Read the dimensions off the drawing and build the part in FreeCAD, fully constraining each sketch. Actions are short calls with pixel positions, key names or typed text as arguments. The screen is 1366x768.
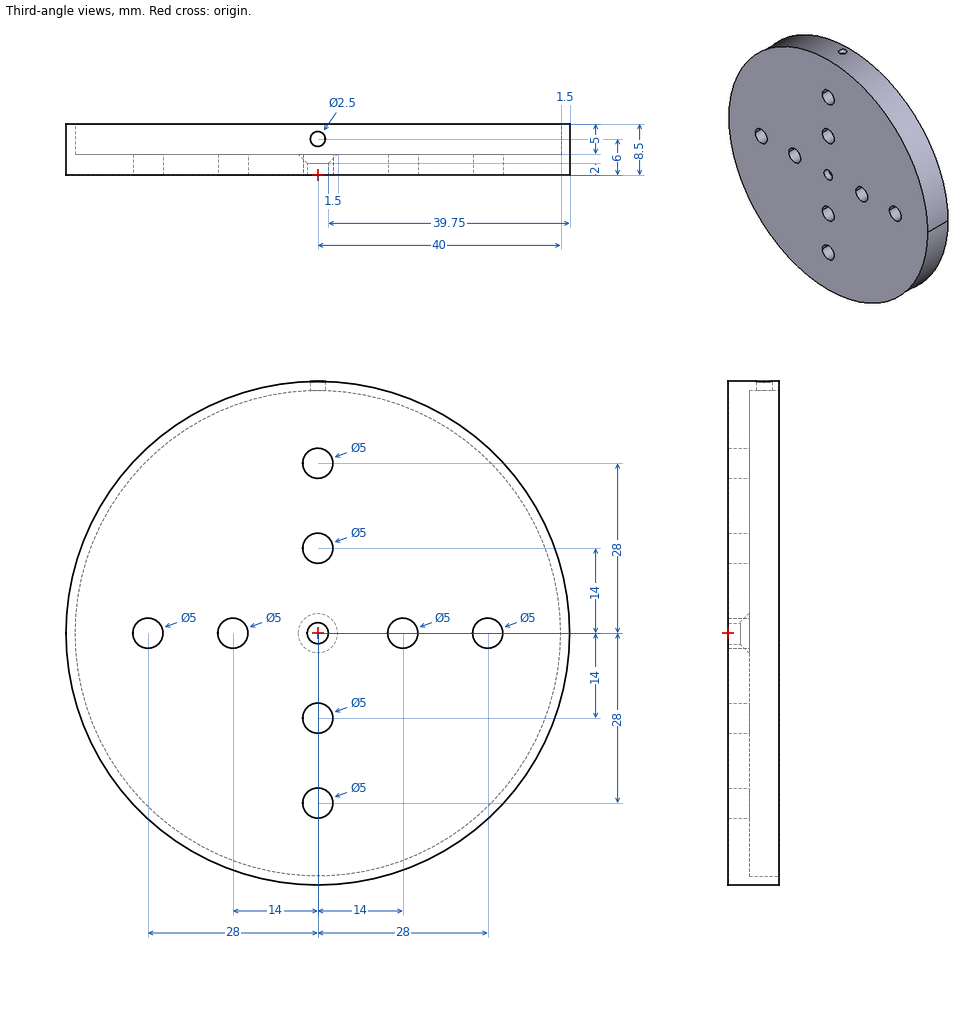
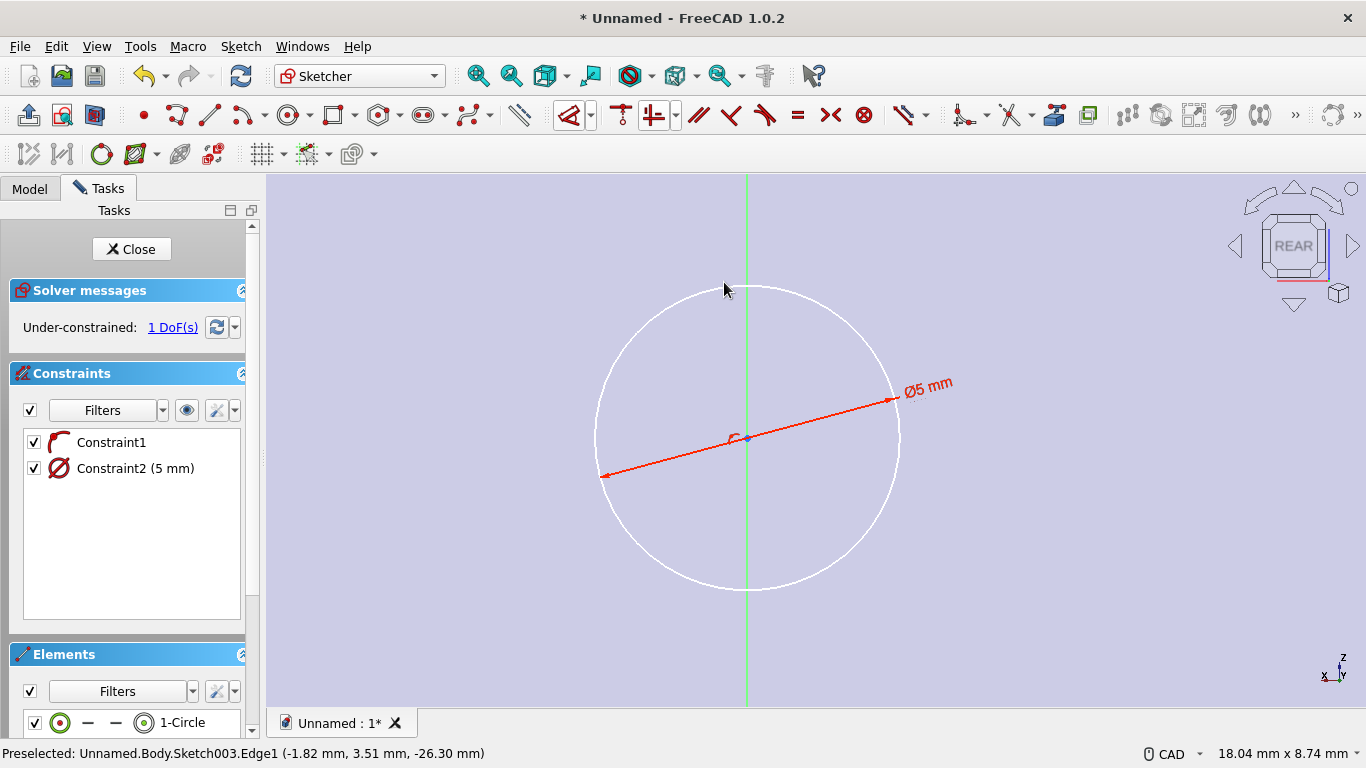
click(747, 438)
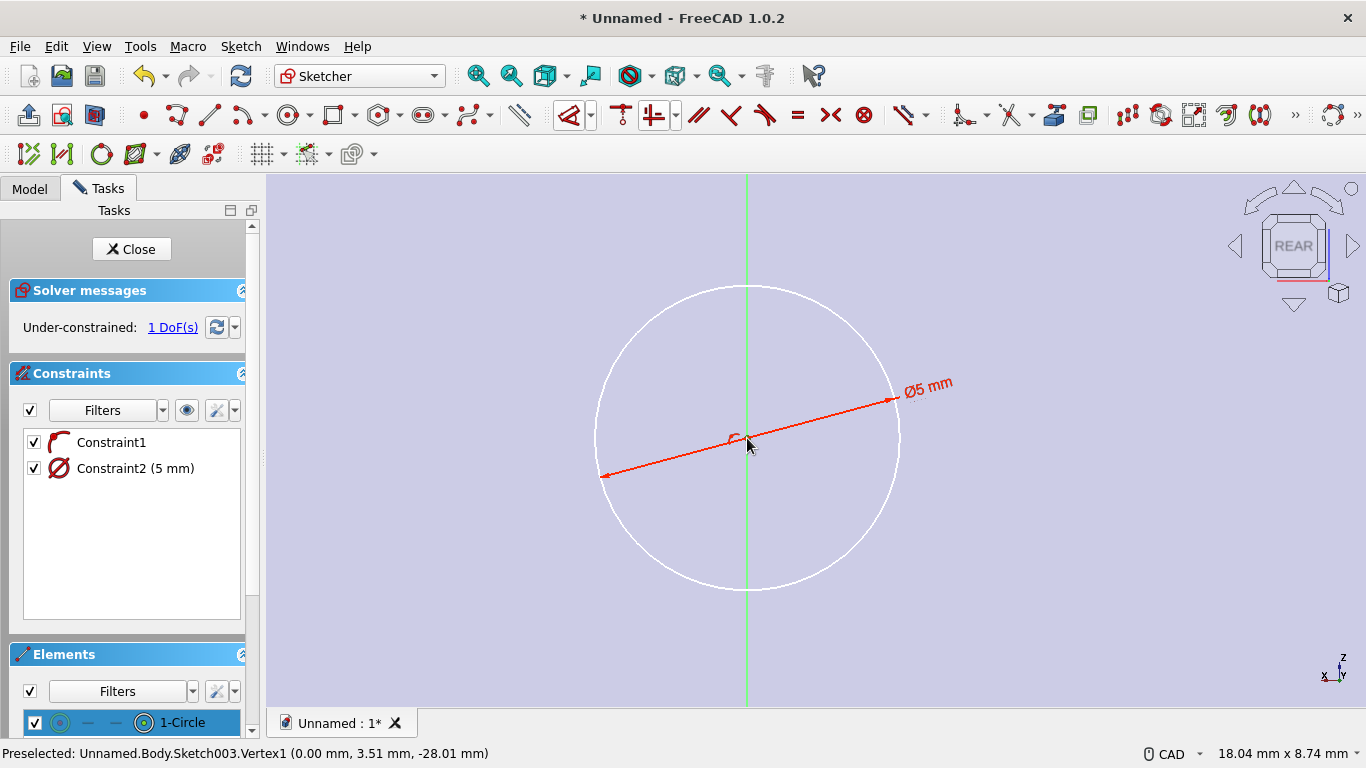
click(590, 116)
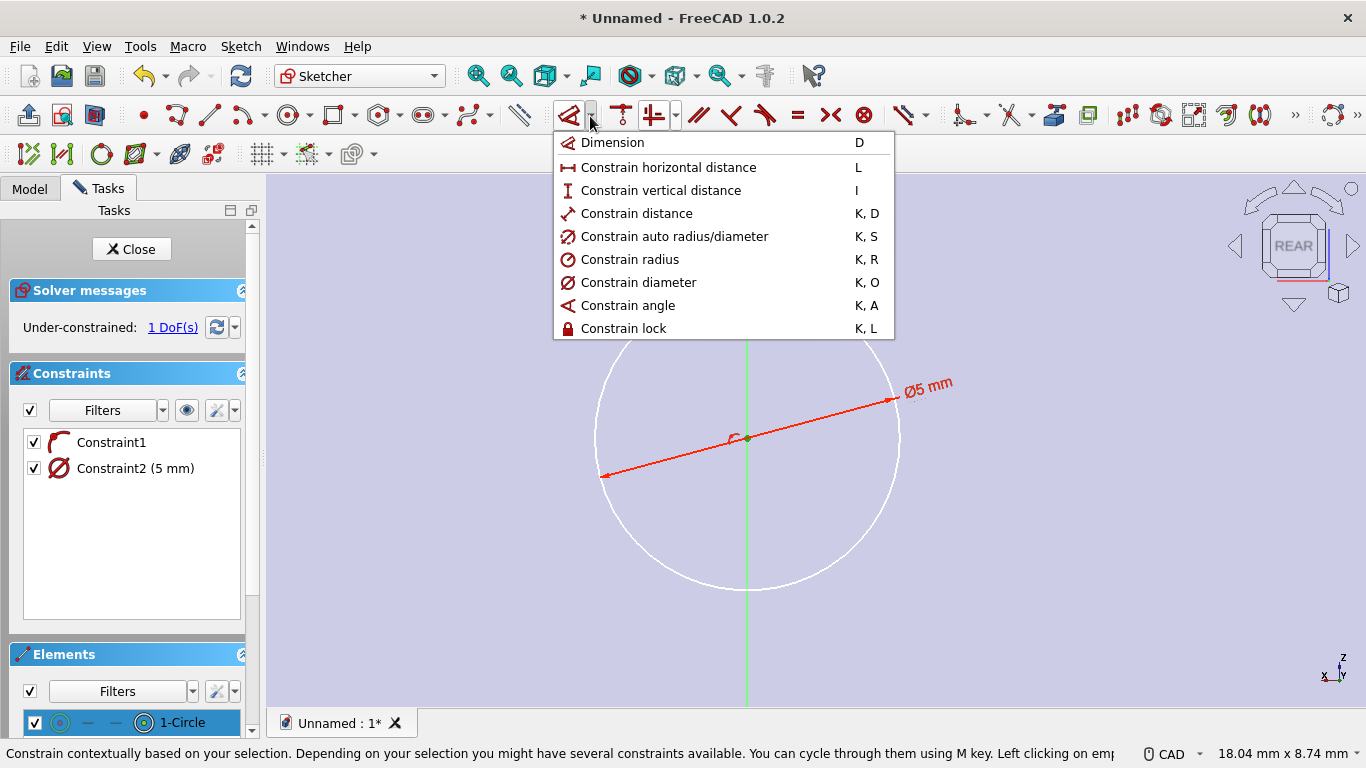
click(724, 190)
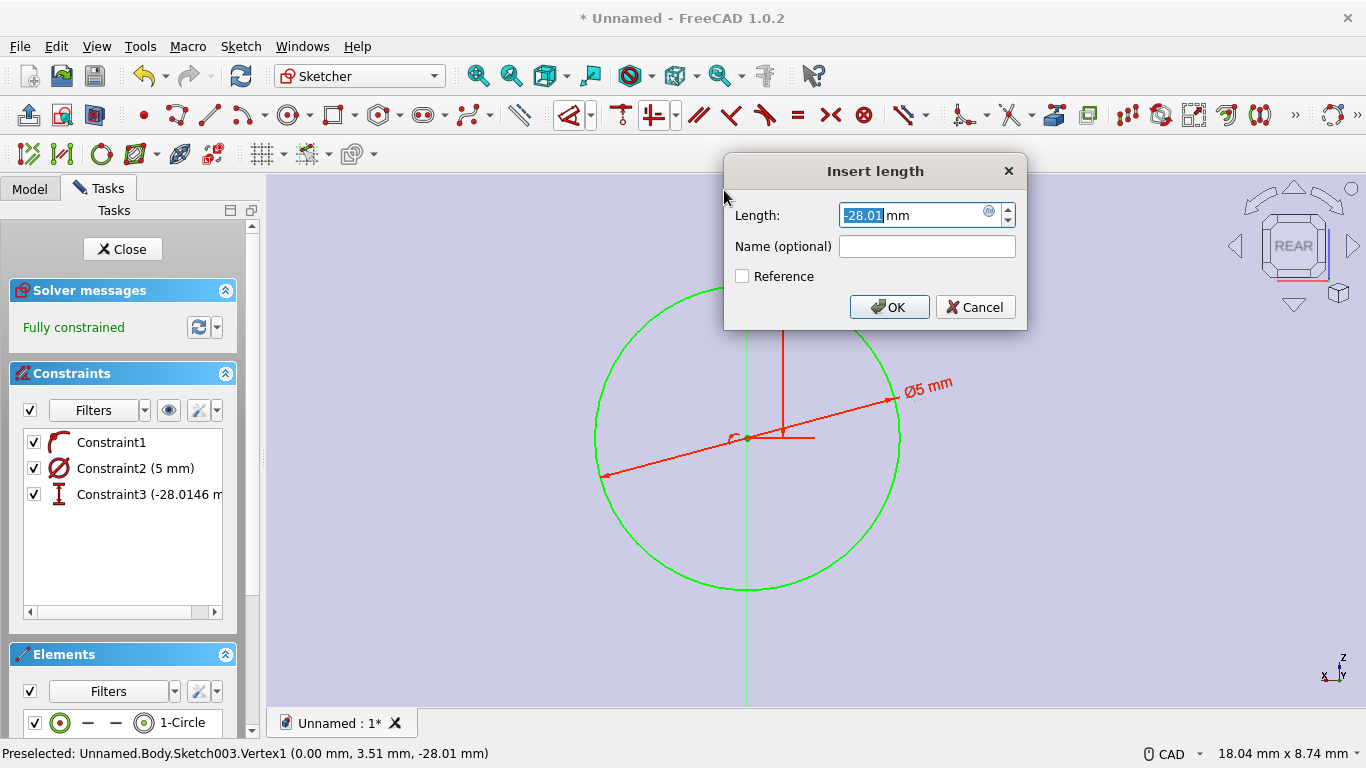
text(-28)
key(Return)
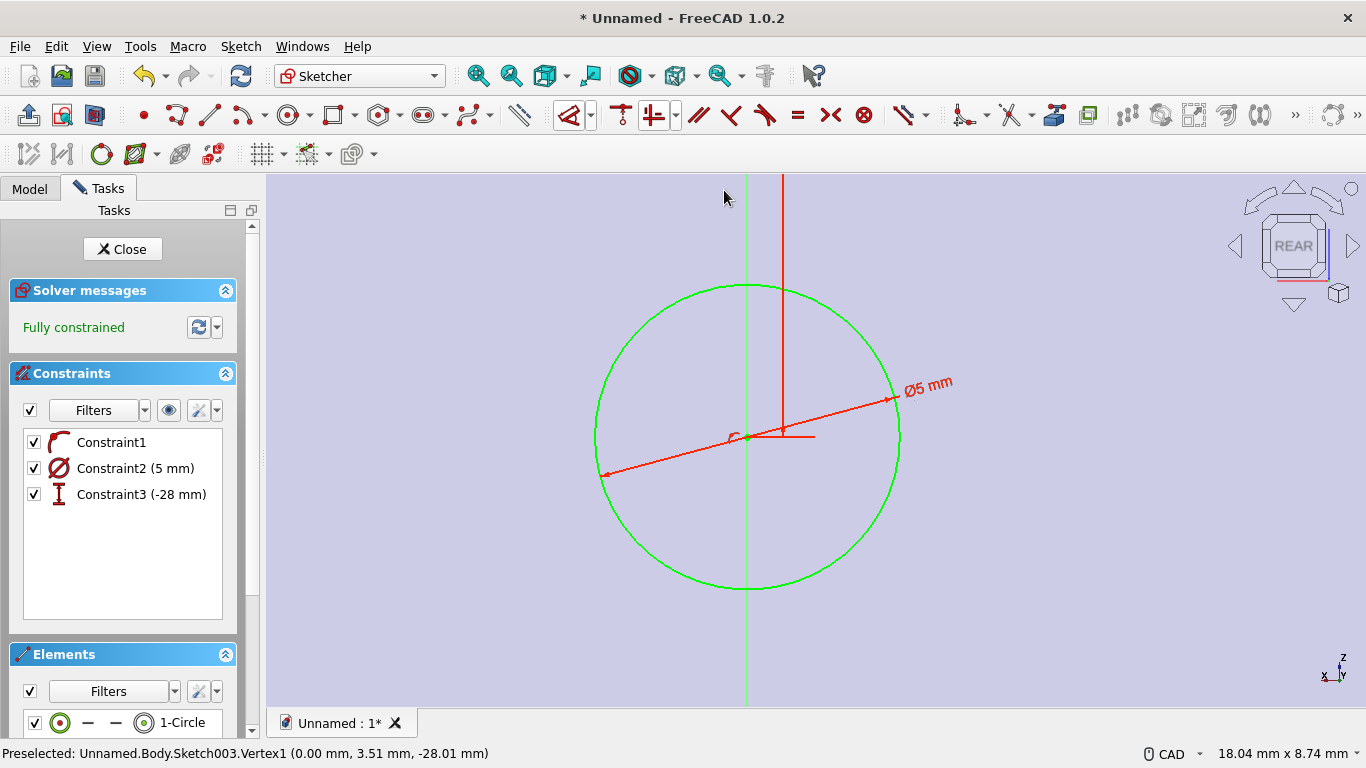
click(123, 249)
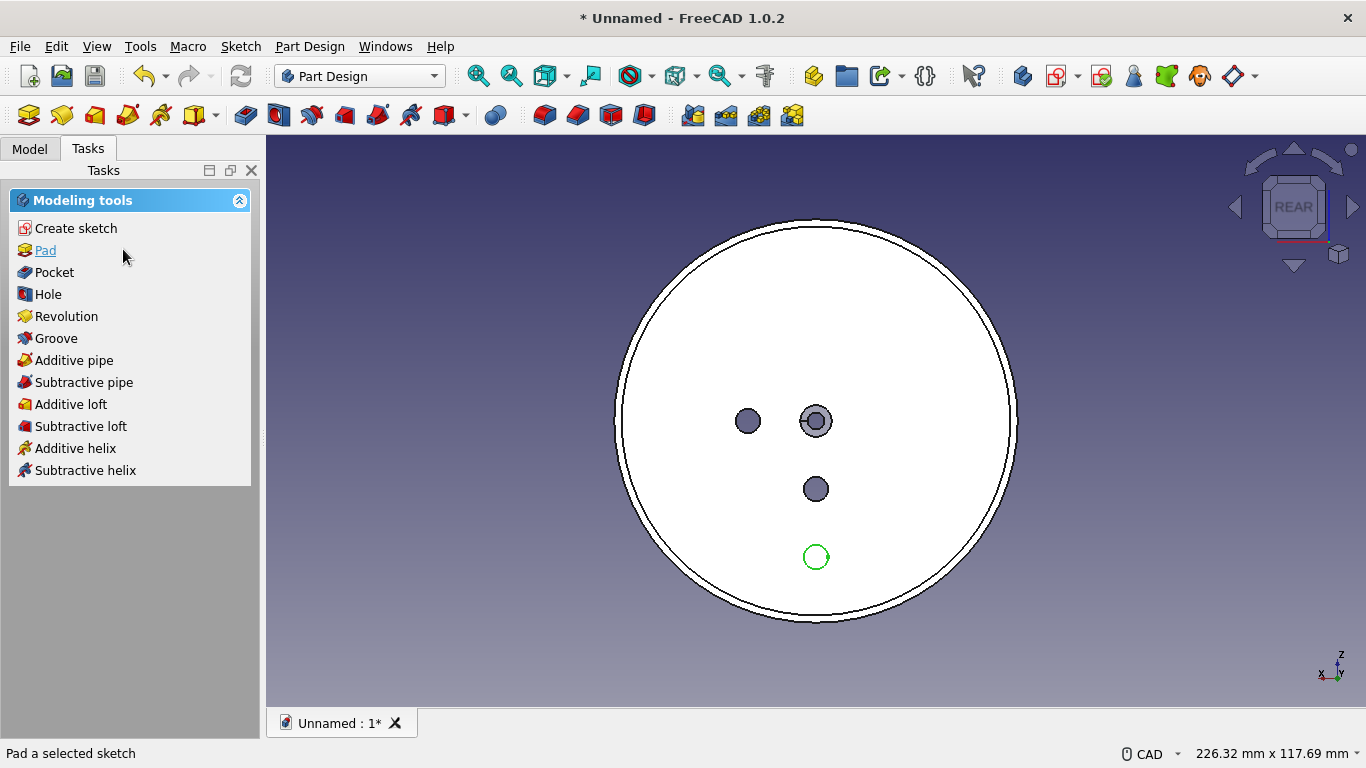
click(246, 116)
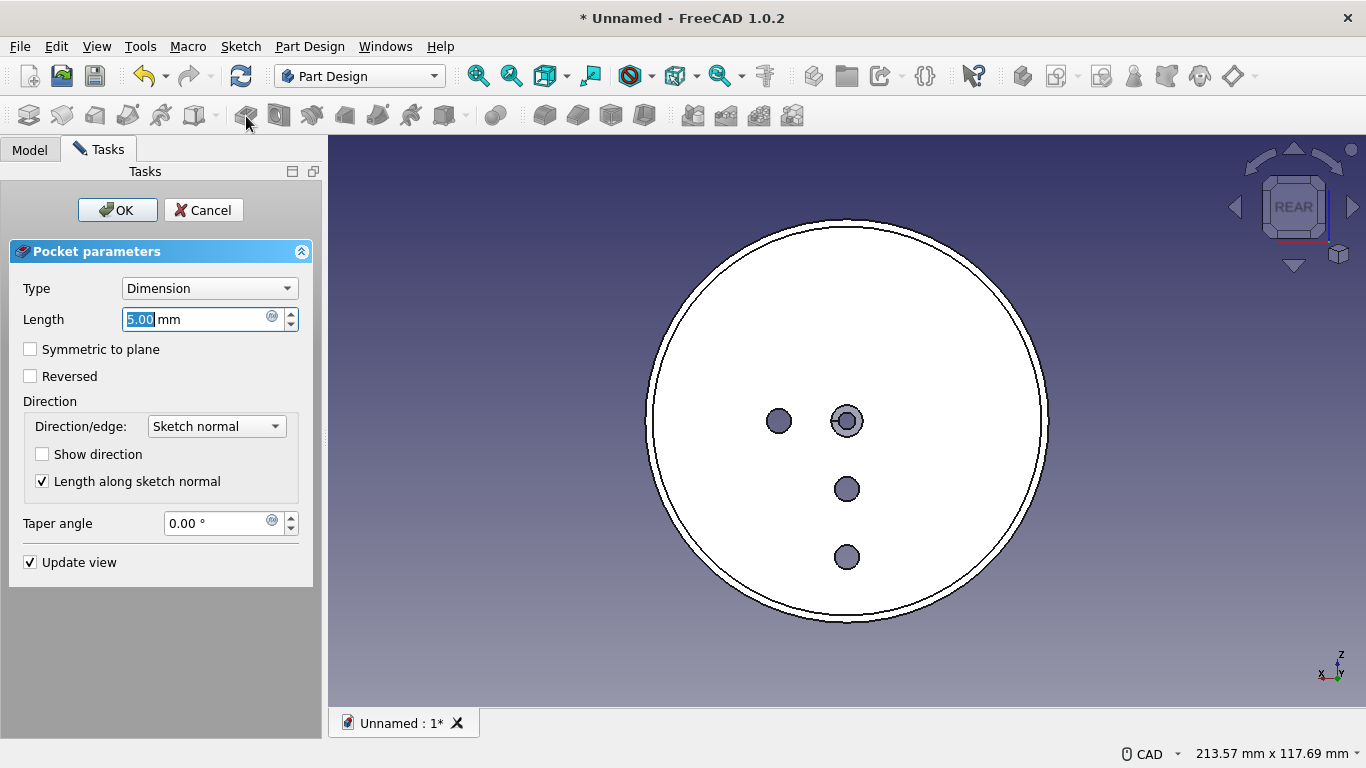
click(210, 288)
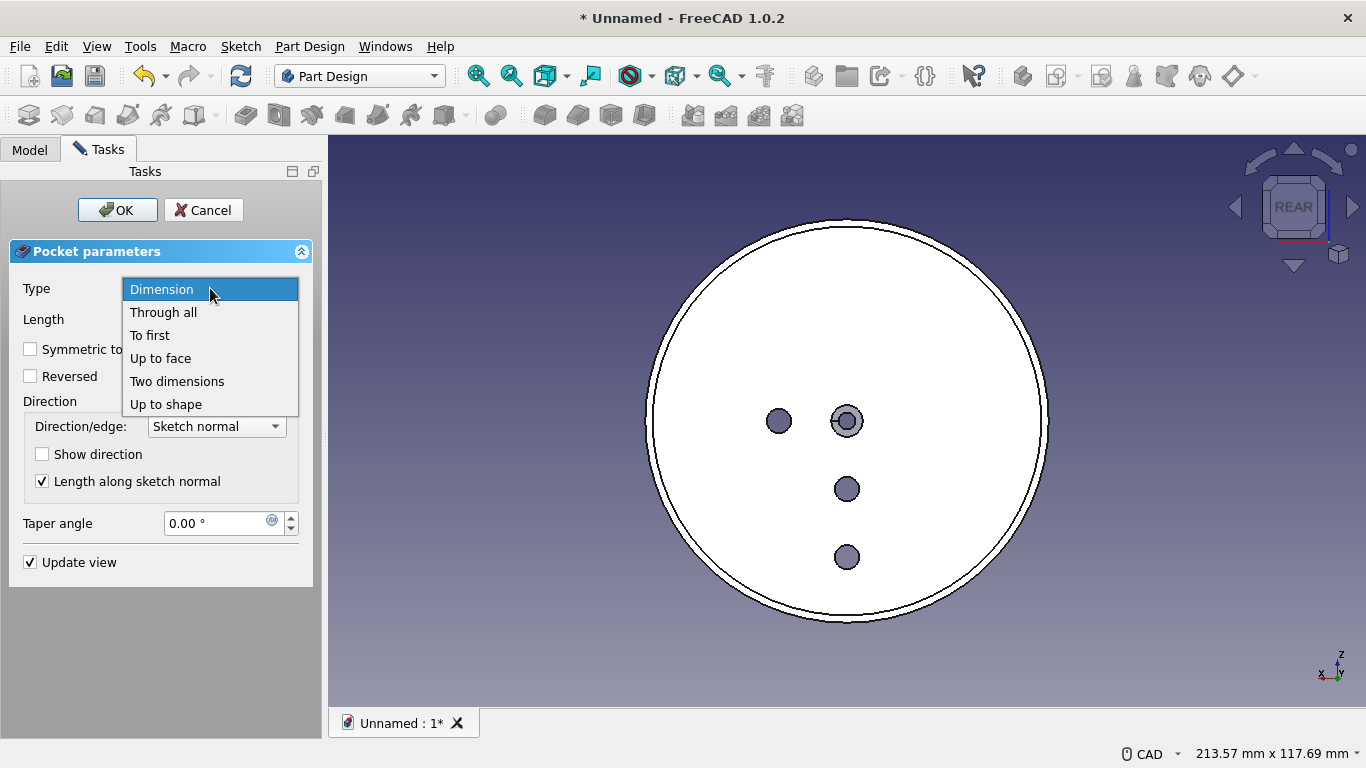
click(208, 336)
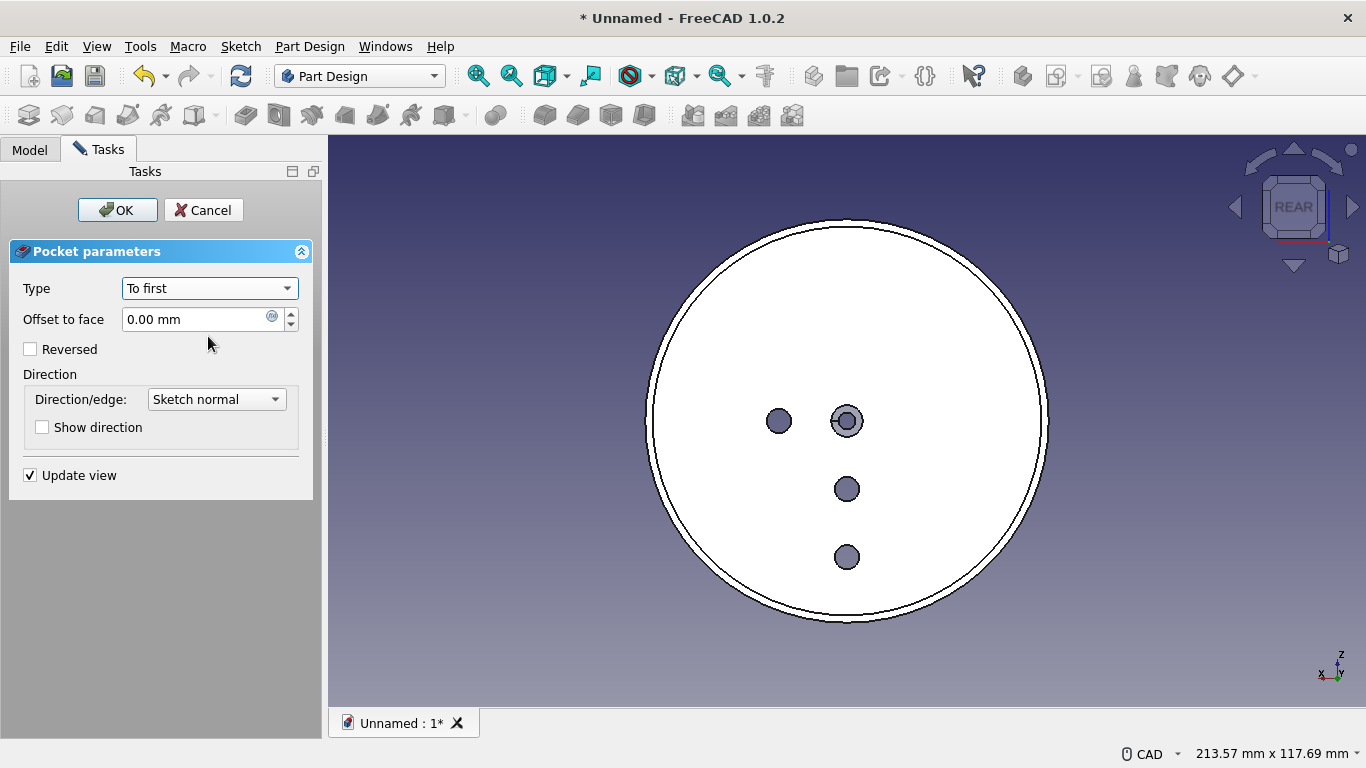
click(118, 210)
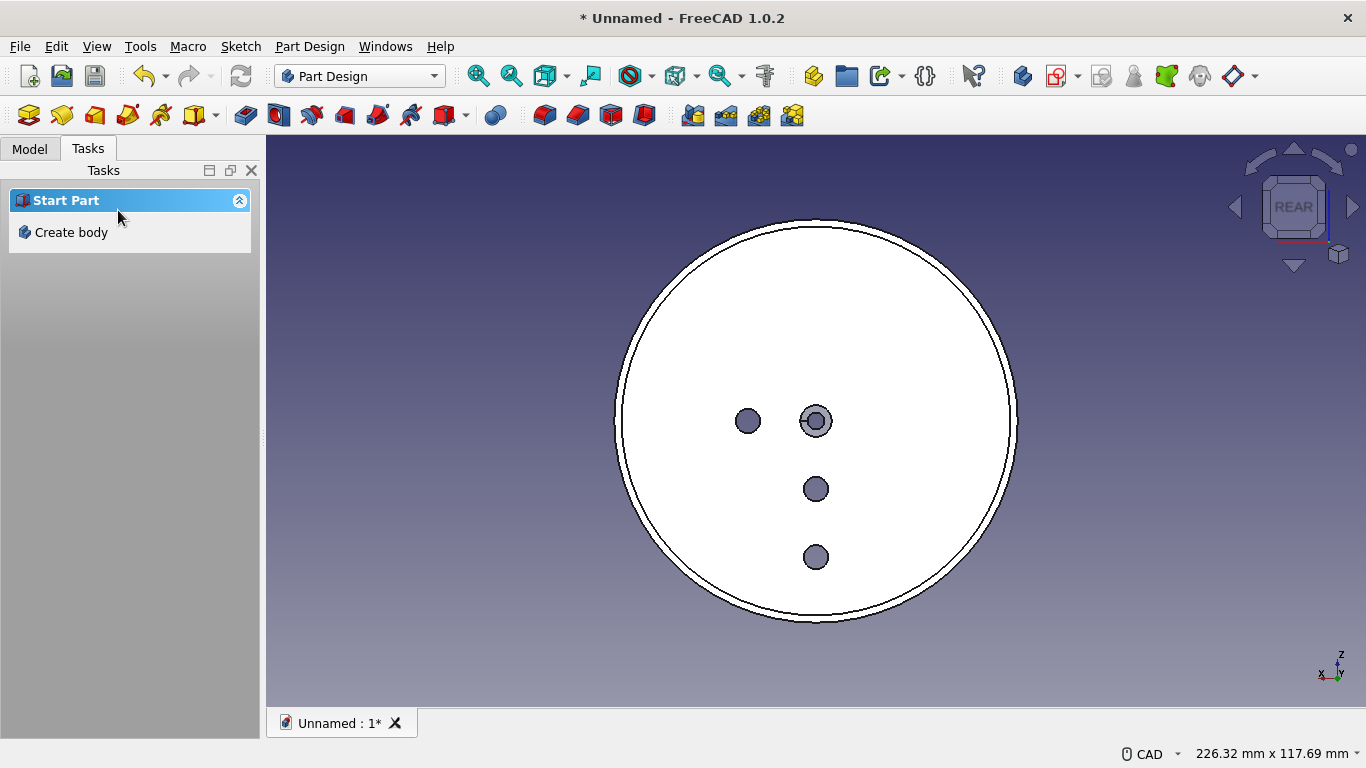
click(816, 309)